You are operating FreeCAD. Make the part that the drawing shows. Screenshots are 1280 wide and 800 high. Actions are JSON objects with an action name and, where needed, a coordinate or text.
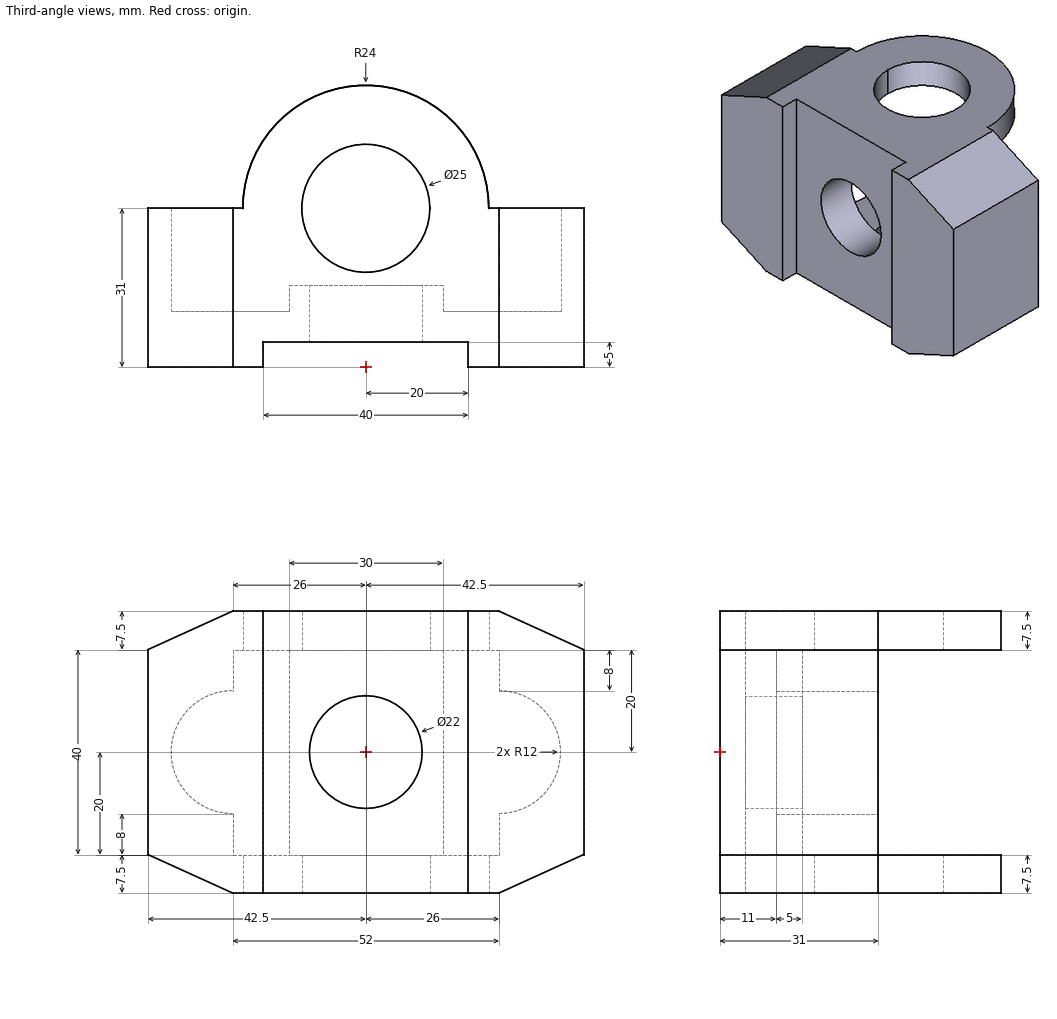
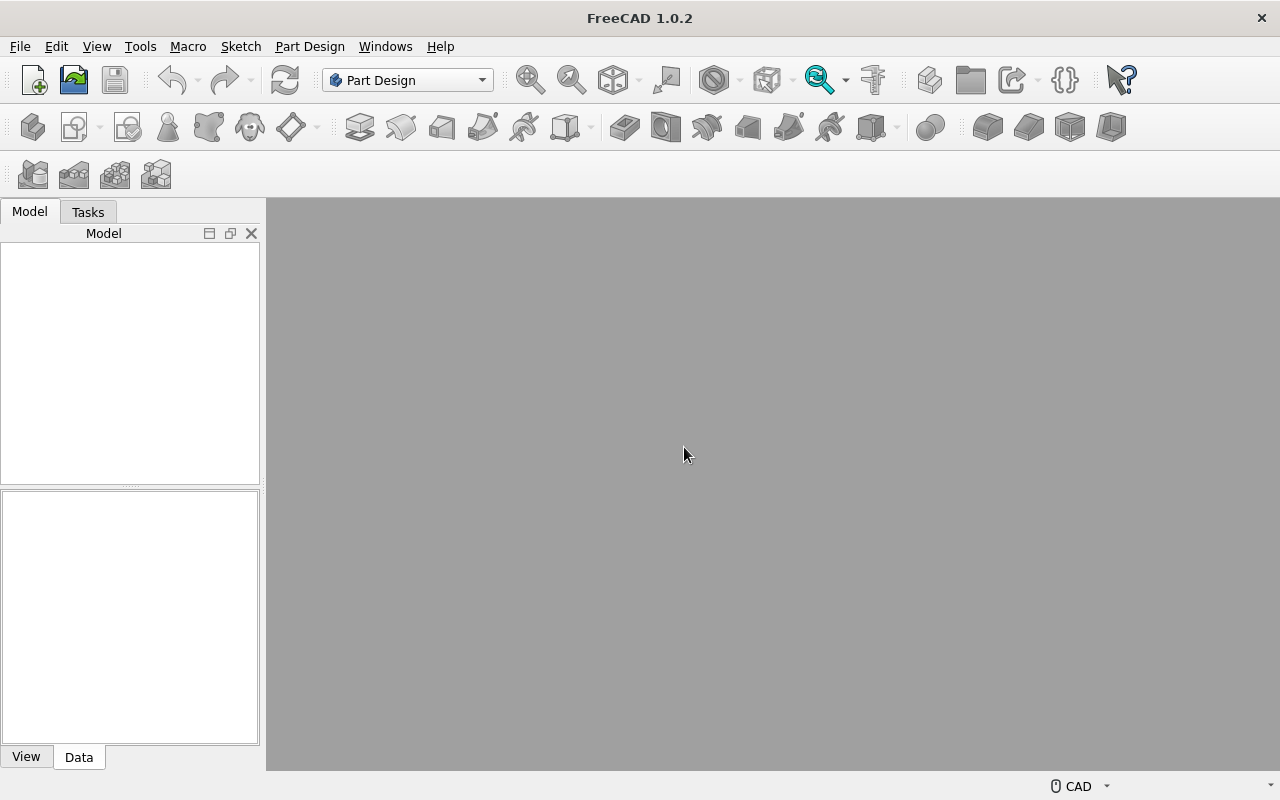
{"action": "left_click", "coordinate": [33, 80]}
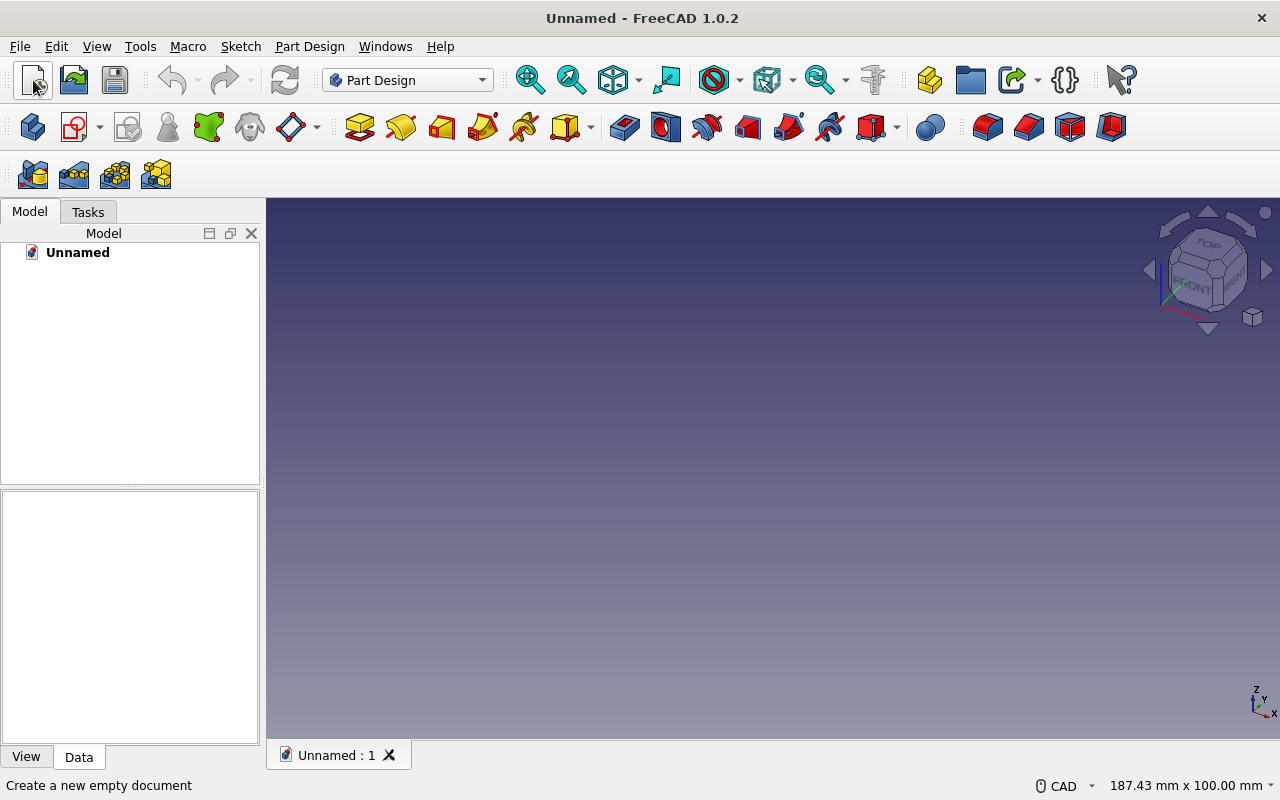
{"action": "left_click", "coordinate": [74, 128]}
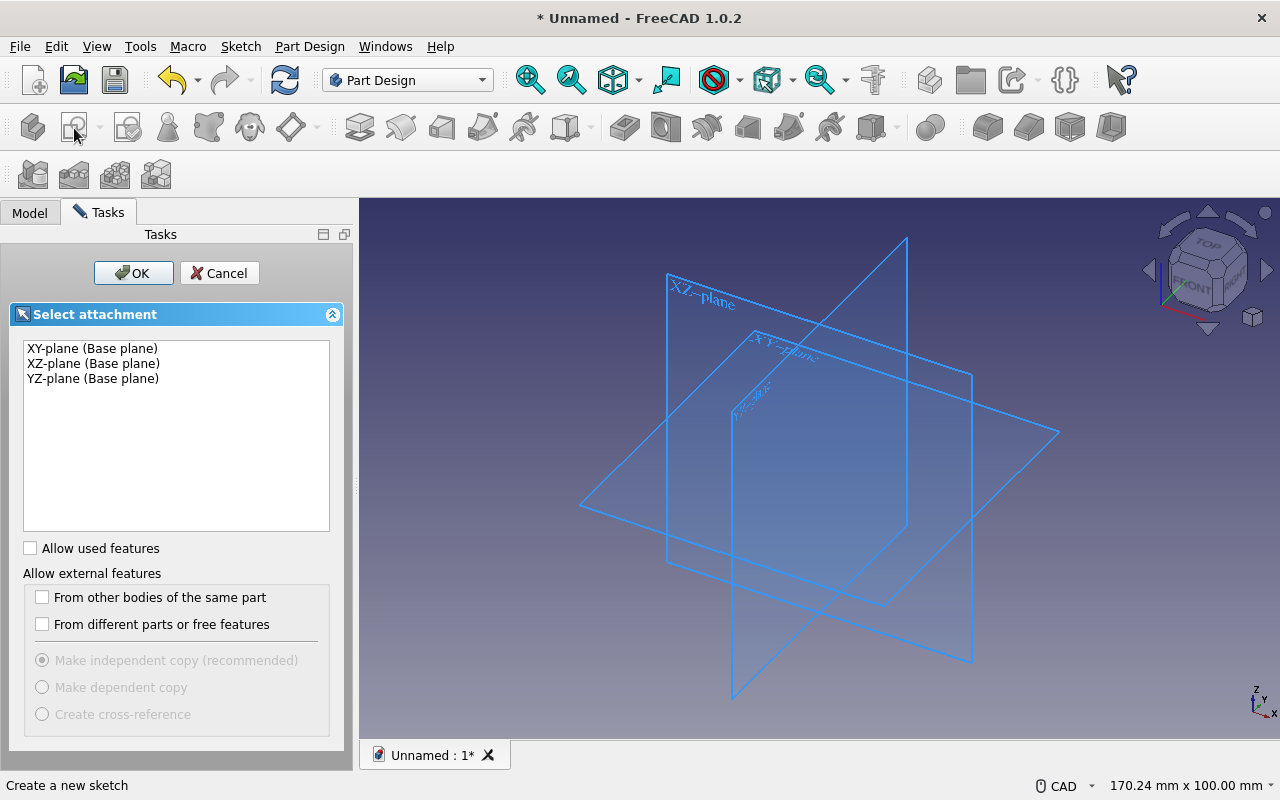
{"action": "left_click", "coordinate": [84, 364]}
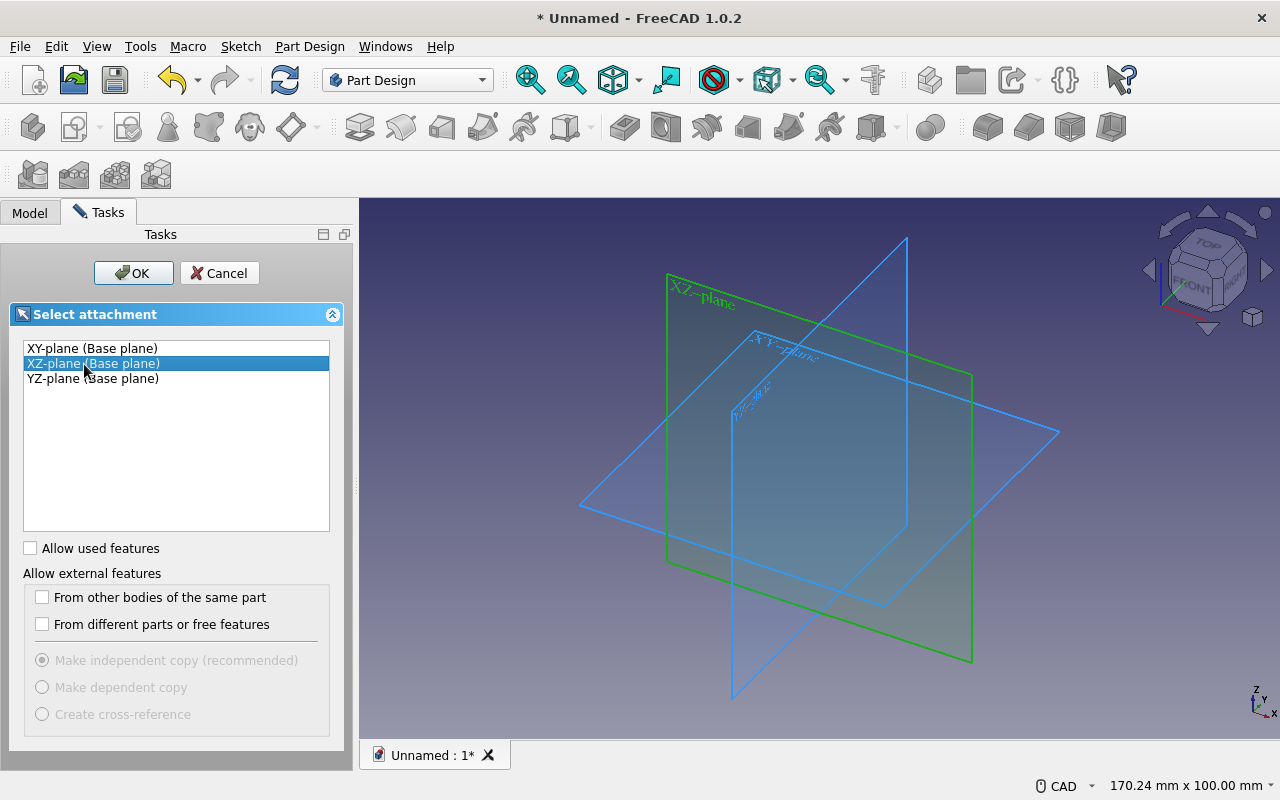
{"action": "left_click", "coordinate": [134, 273]}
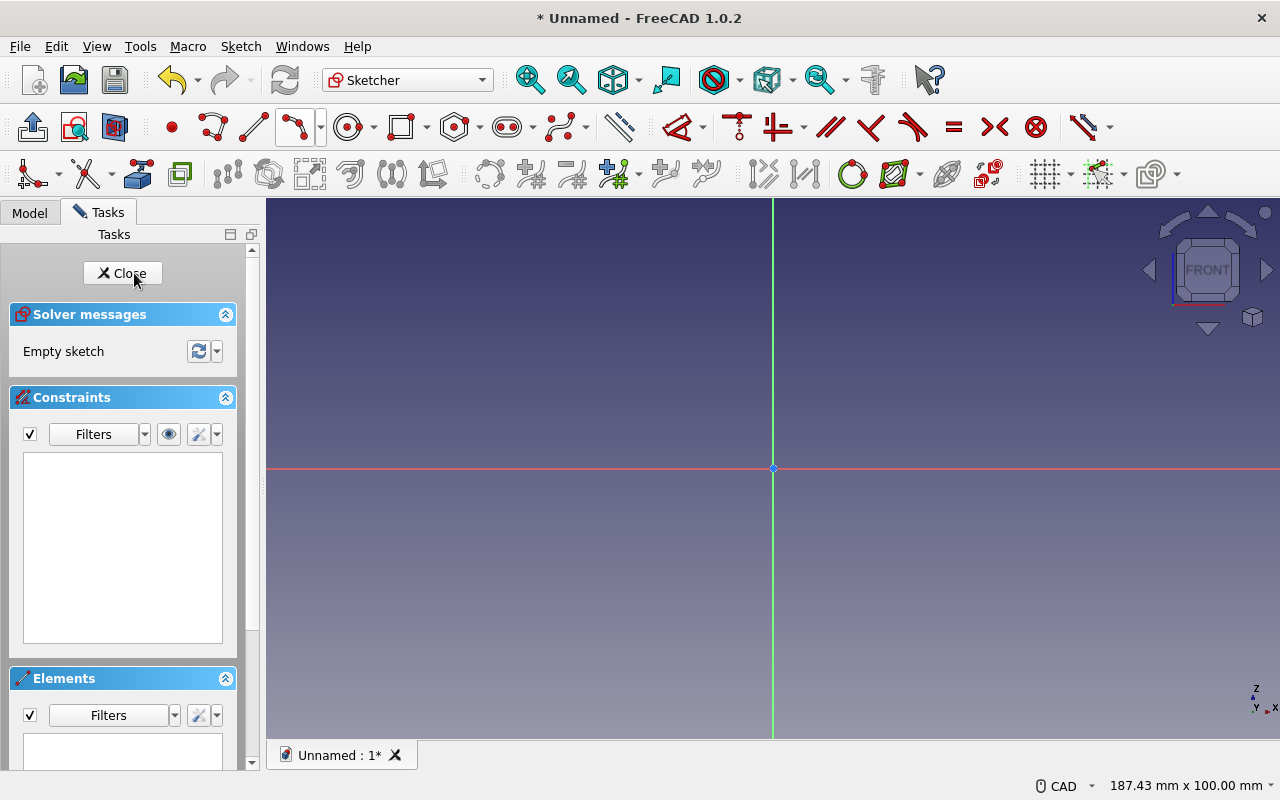
{"action": "left_click", "coordinate": [213, 128]}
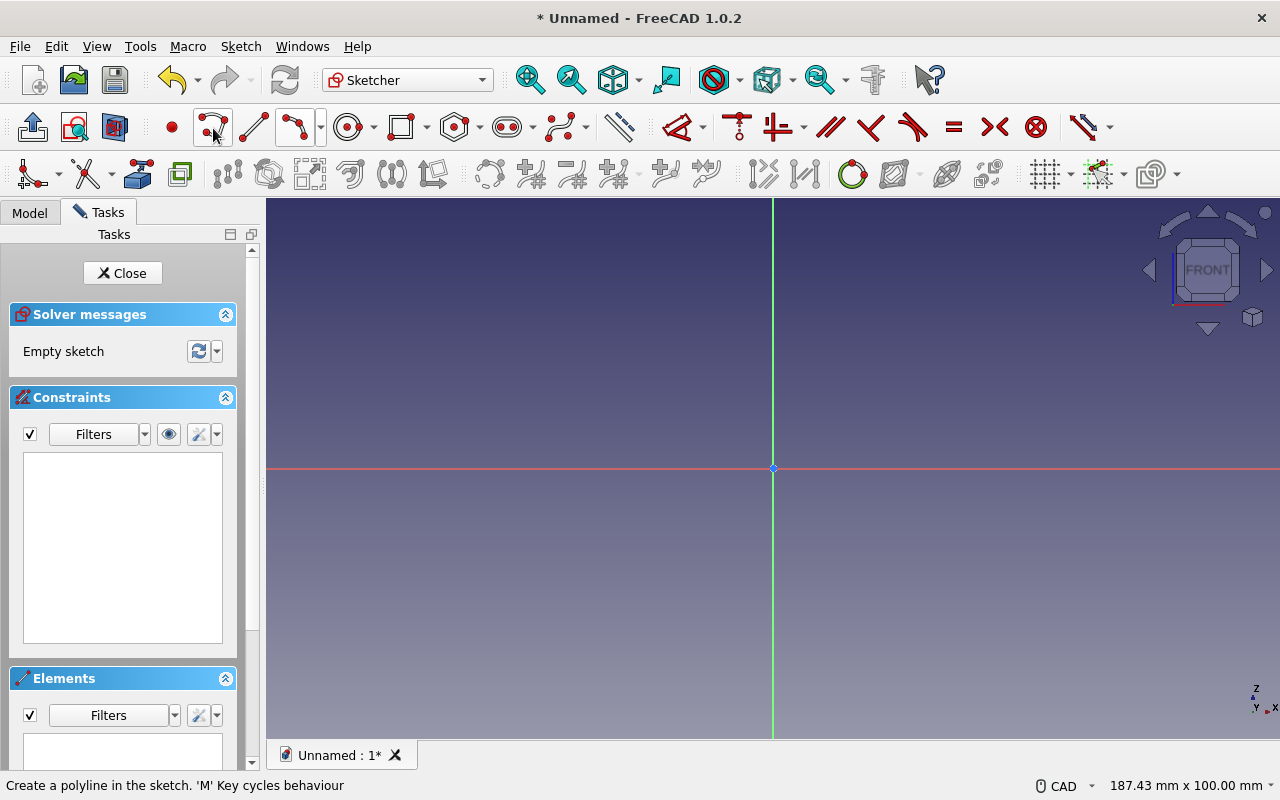
{"action": "left_click", "coordinate": [914, 617]}
{"action": "left_click", "coordinate": [632, 617]}
{"action": "left_click", "coordinate": [543, 577]}
{"action": "left_click", "coordinate": [543, 360]}
{"action": "left_click", "coordinate": [632, 320]}
{"action": "left_click", "coordinate": [914, 320]}
{"action": "left_click", "coordinate": [1003, 360]}
{"action": "left_click", "coordinate": [1003, 577]}
{"action": "left_click", "coordinate": [914, 618]}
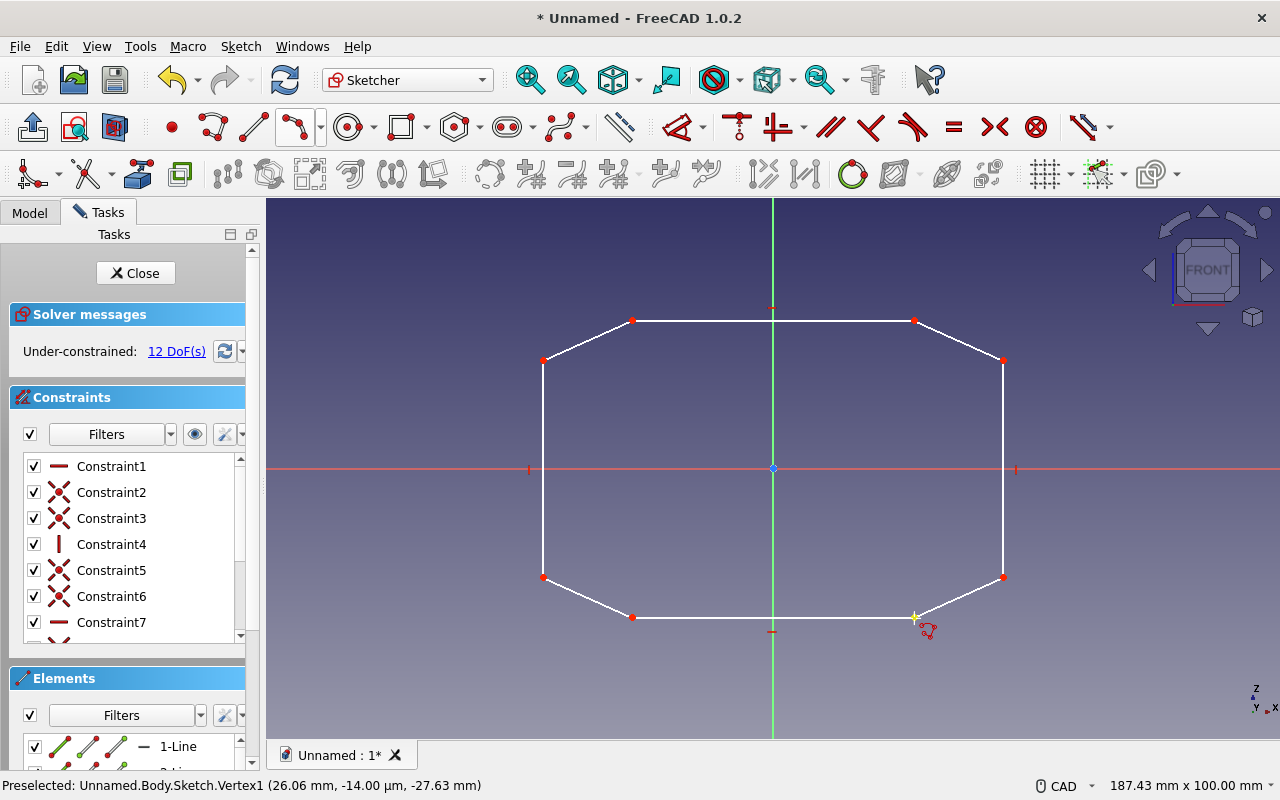
{"action": "left_click", "coordinate": [914, 404]}
{"action": "left_click", "coordinate": [914, 360]}
{"action": "left_click", "coordinate": [632, 360]}
{"action": "left_click", "coordinate": [632, 404]}
{"action": "right_click", "coordinate": [632, 404]}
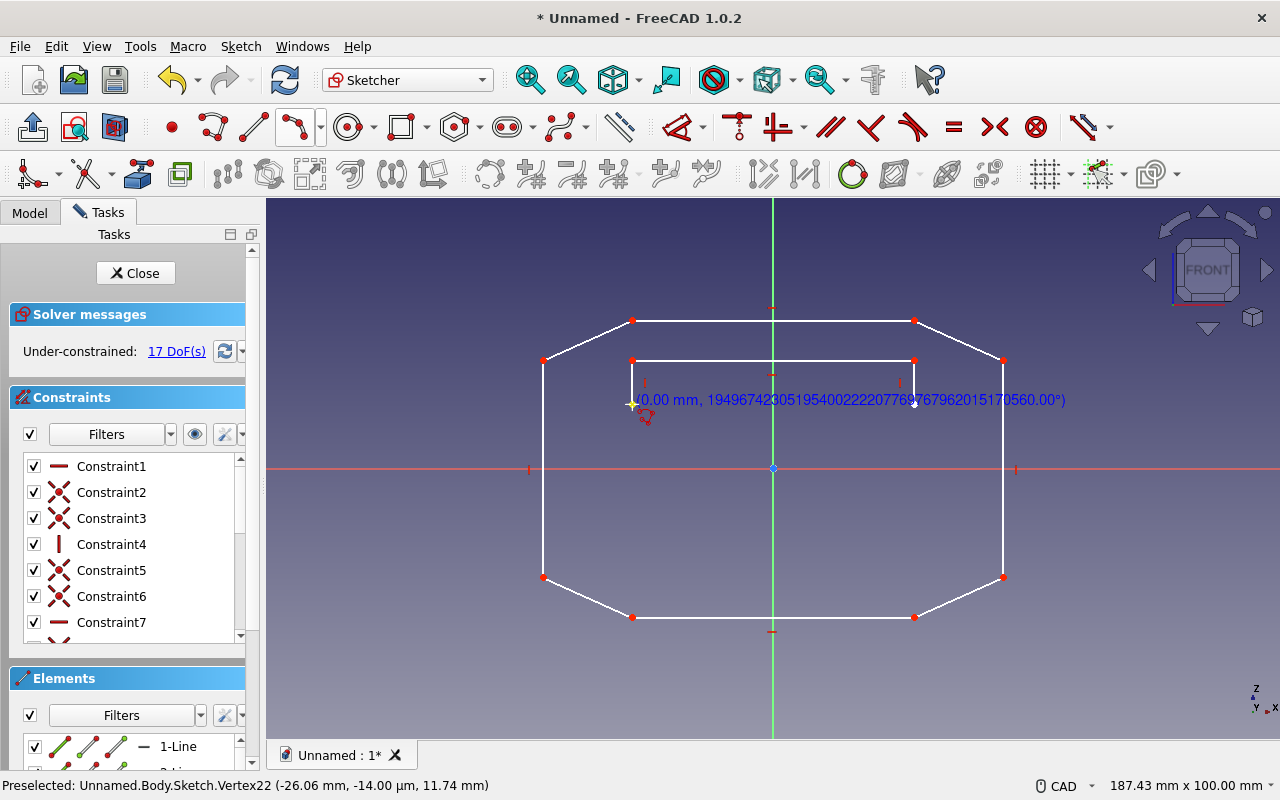
{"action": "left_click", "coordinate": [632, 533]}
{"action": "left_click", "coordinate": [632, 577]}
{"action": "left_click", "coordinate": [914, 577]}
{"action": "left_click", "coordinate": [914, 533]}
{"action": "right_click", "coordinate": [914, 533]}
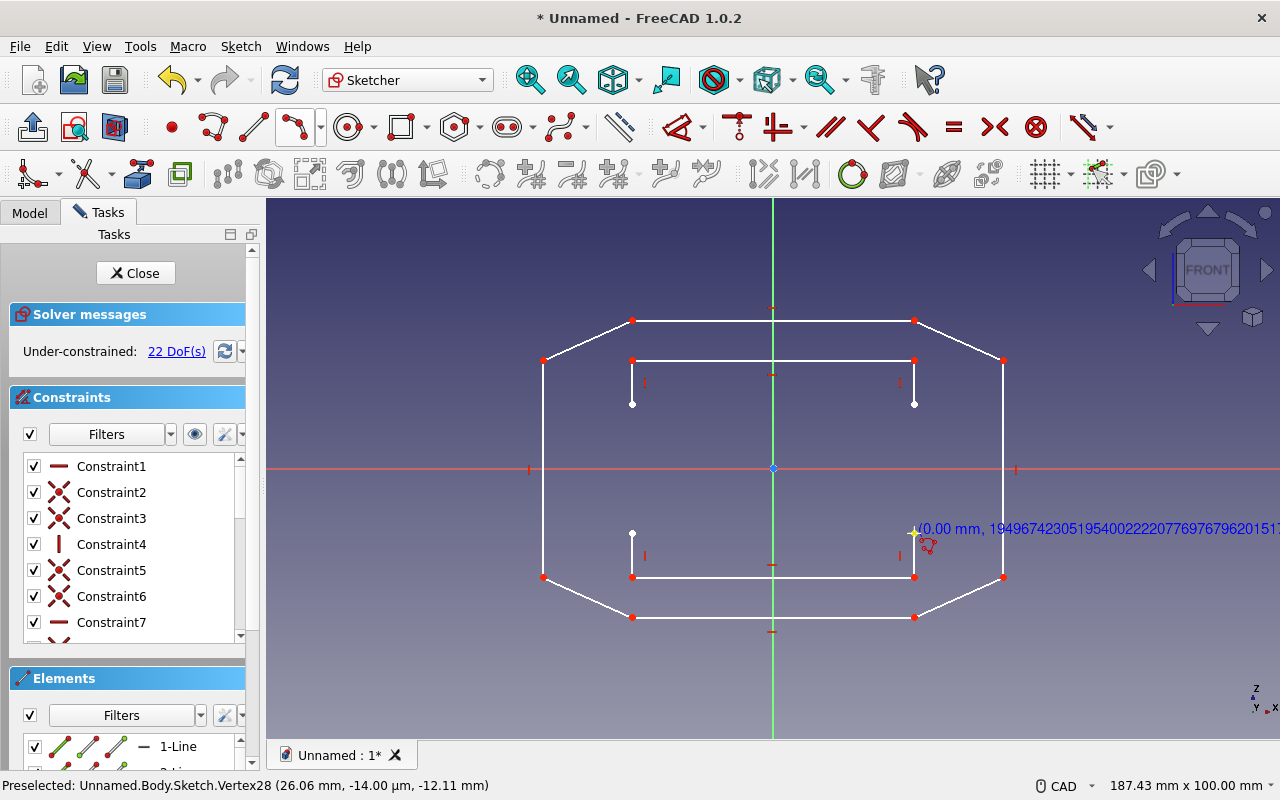
{"action": "left_click", "coordinate": [294, 128]}